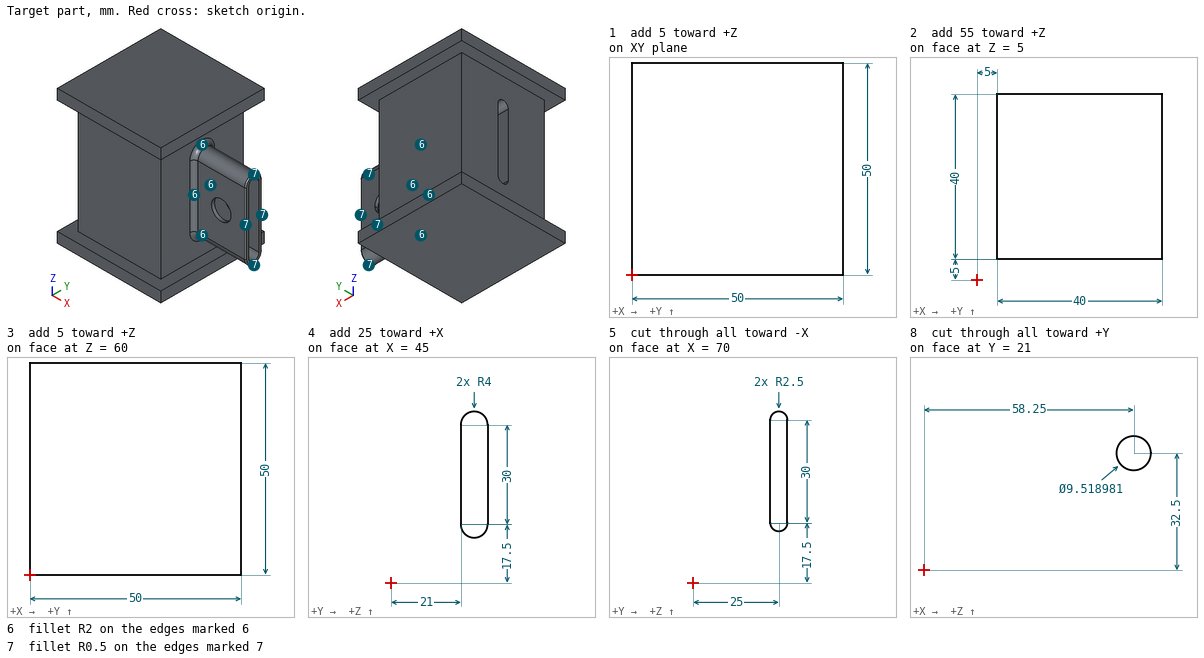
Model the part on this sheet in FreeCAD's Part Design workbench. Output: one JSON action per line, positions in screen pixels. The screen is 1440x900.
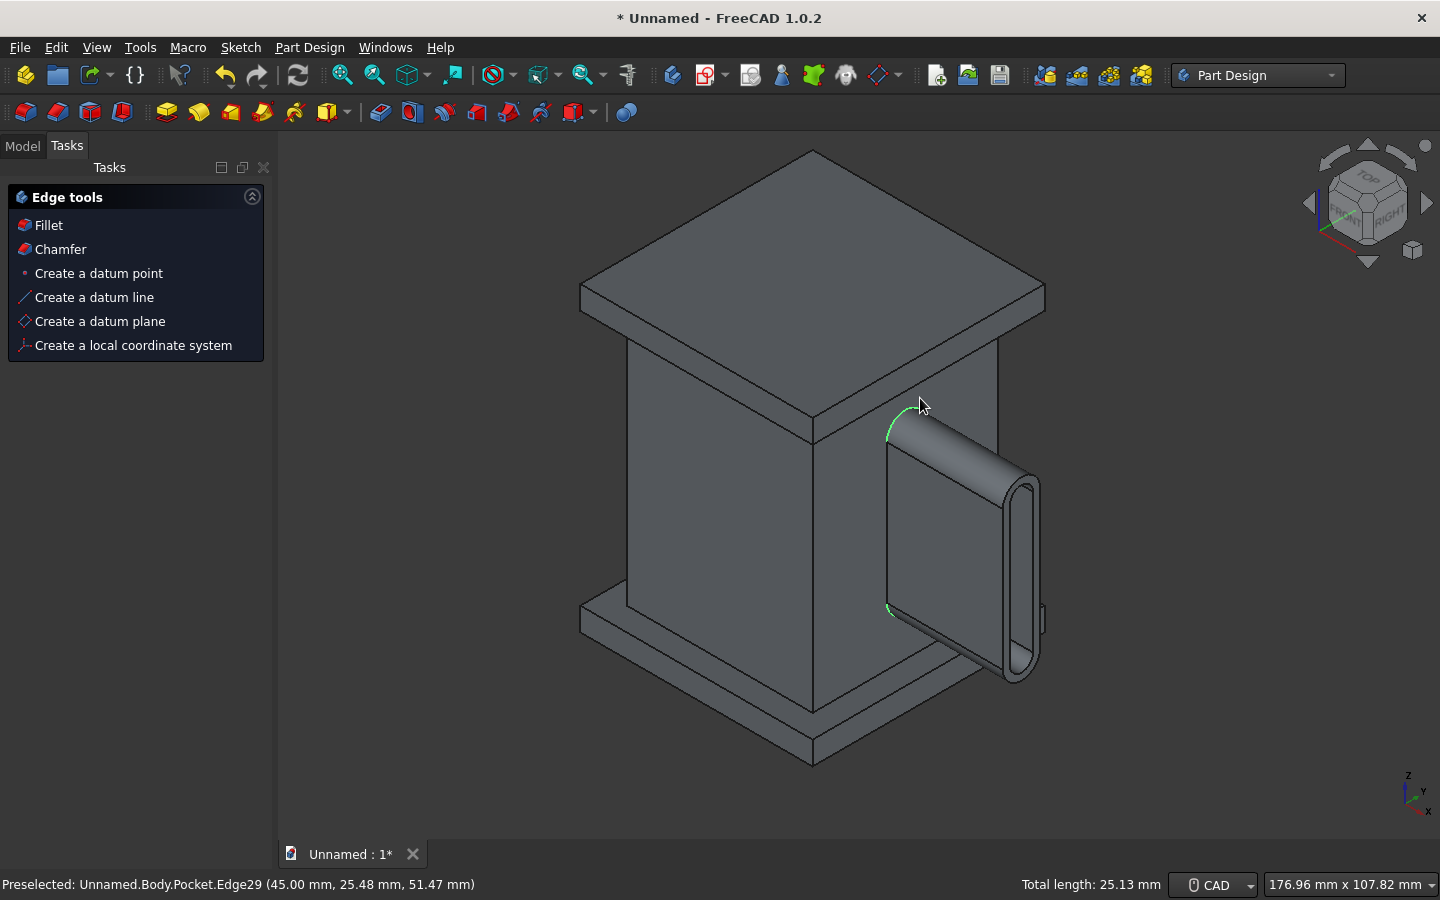
{"action": "key", "text": "2"}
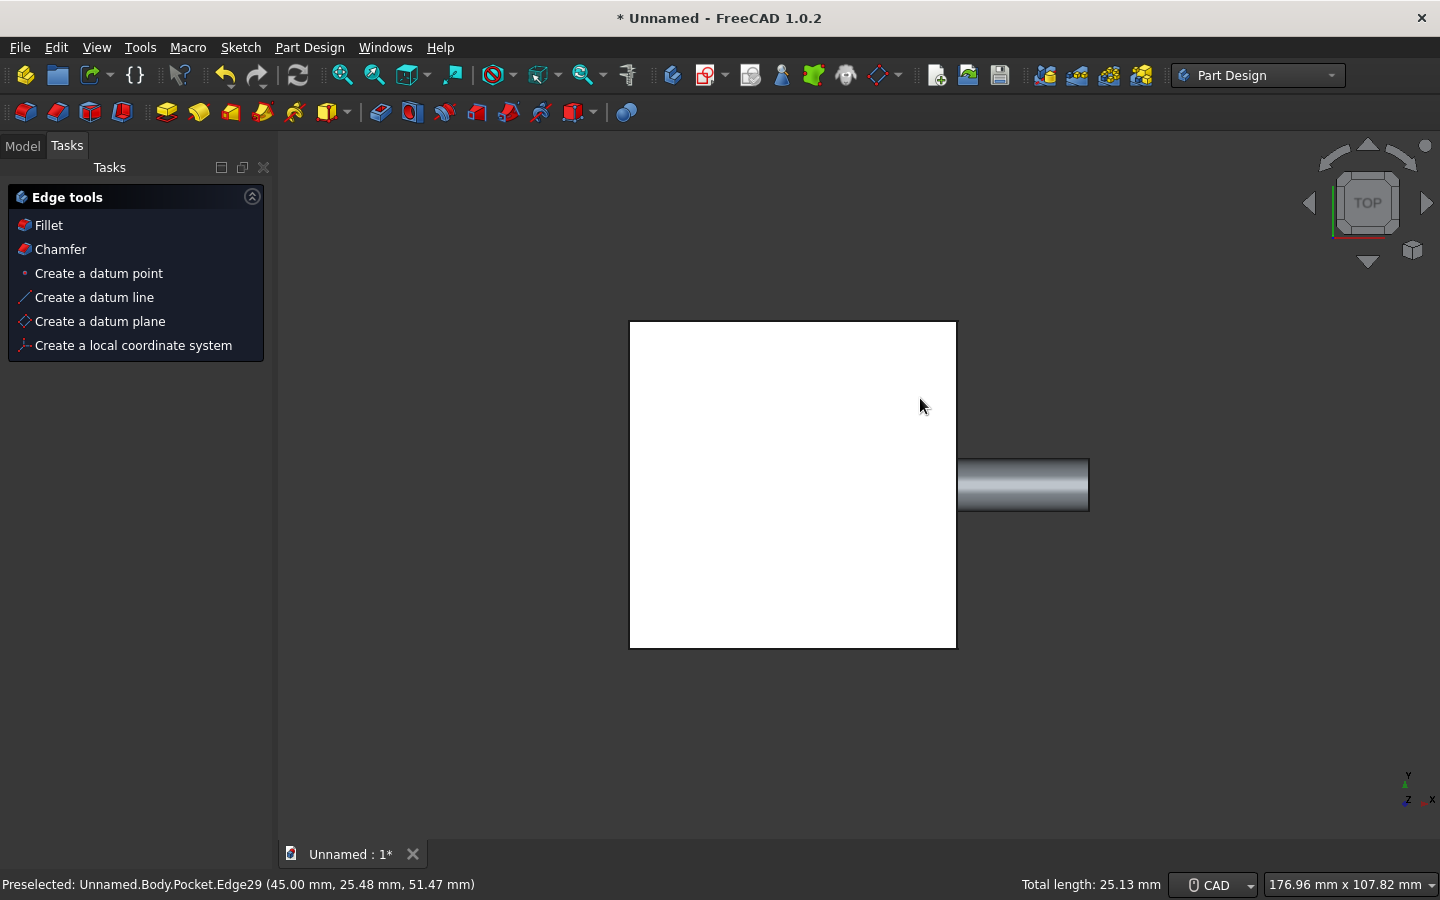
{"action": "key", "text": "1"}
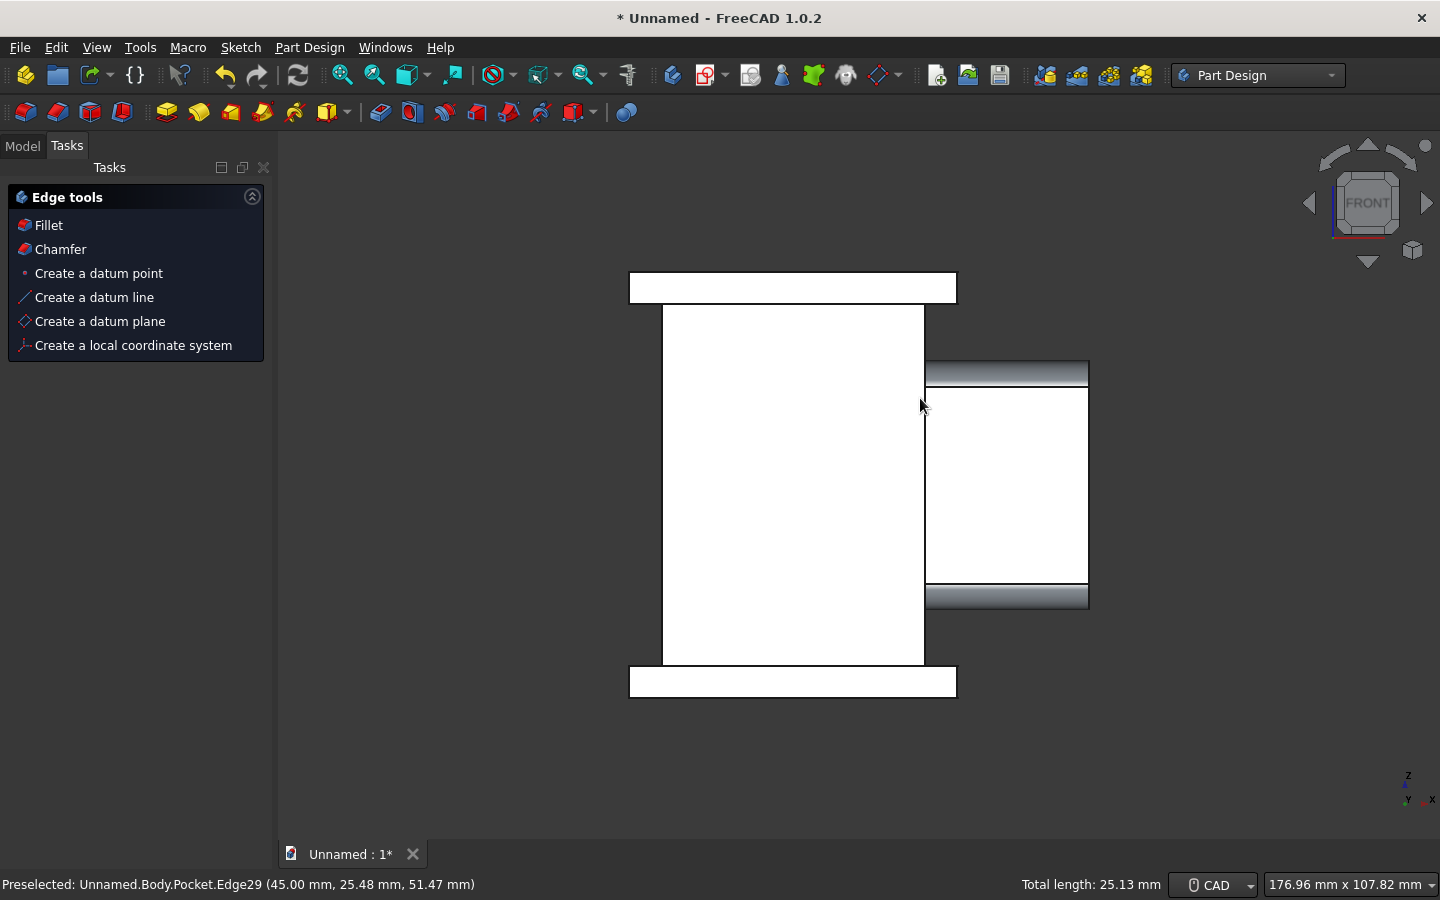
{"action": "key", "text": "3"}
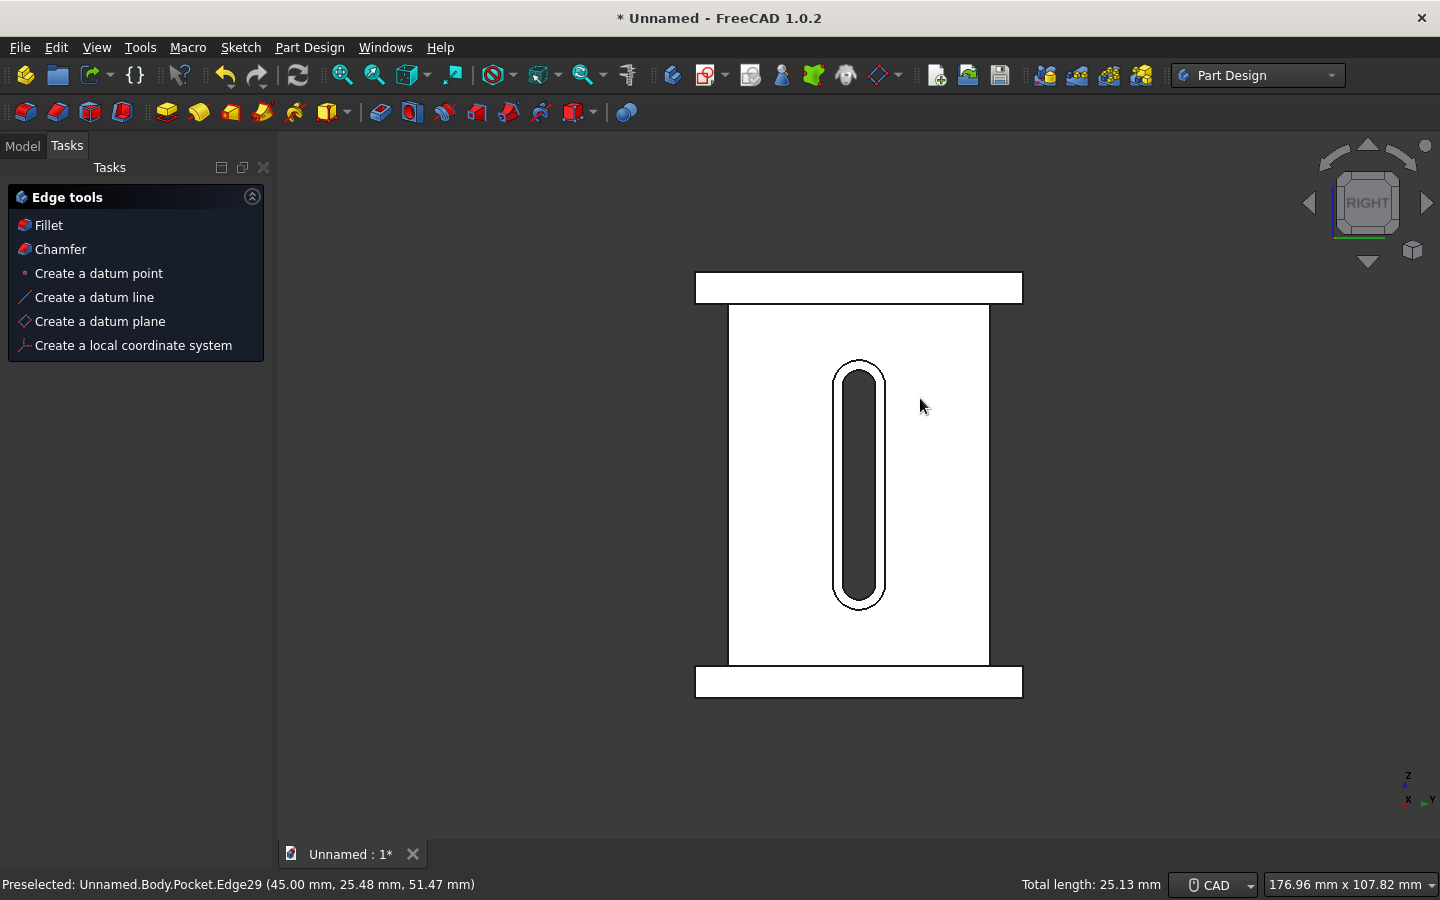
{"action": "key", "text": "5"}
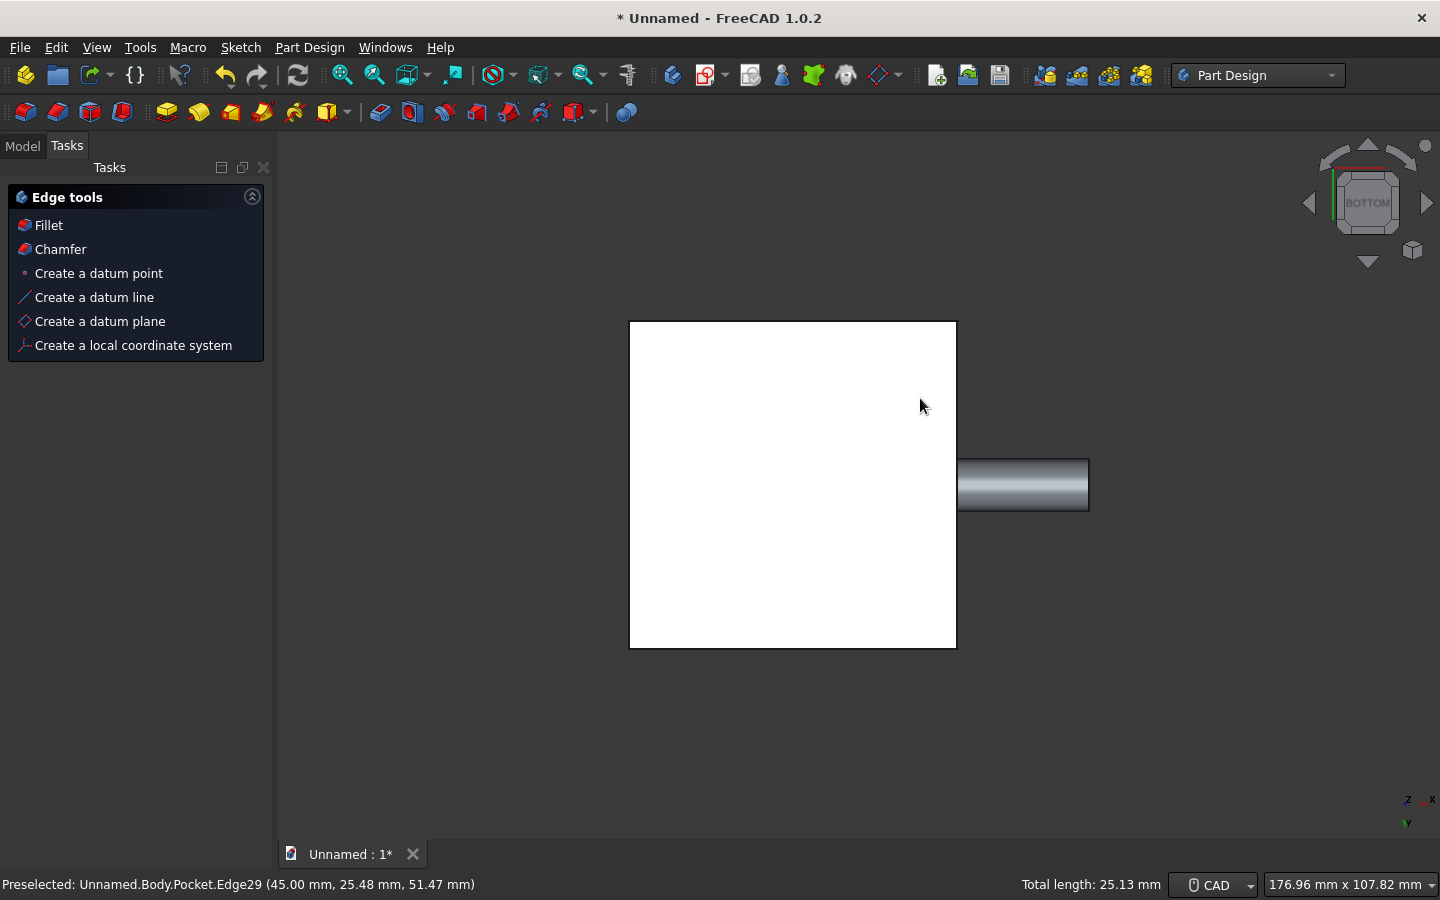
{"action": "key", "text": "4"}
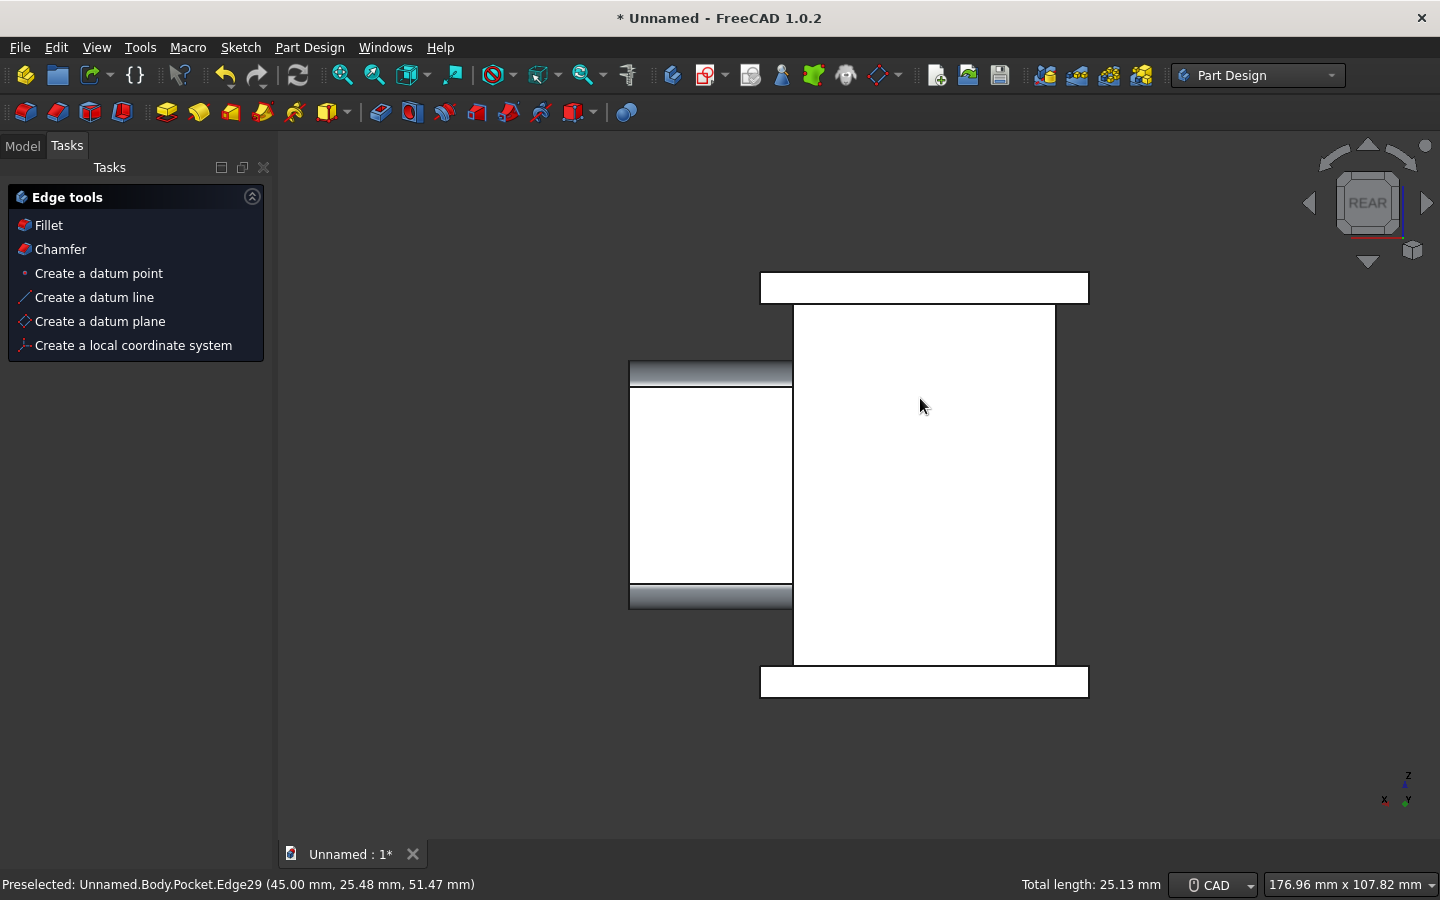
{"action": "key", "text": "6"}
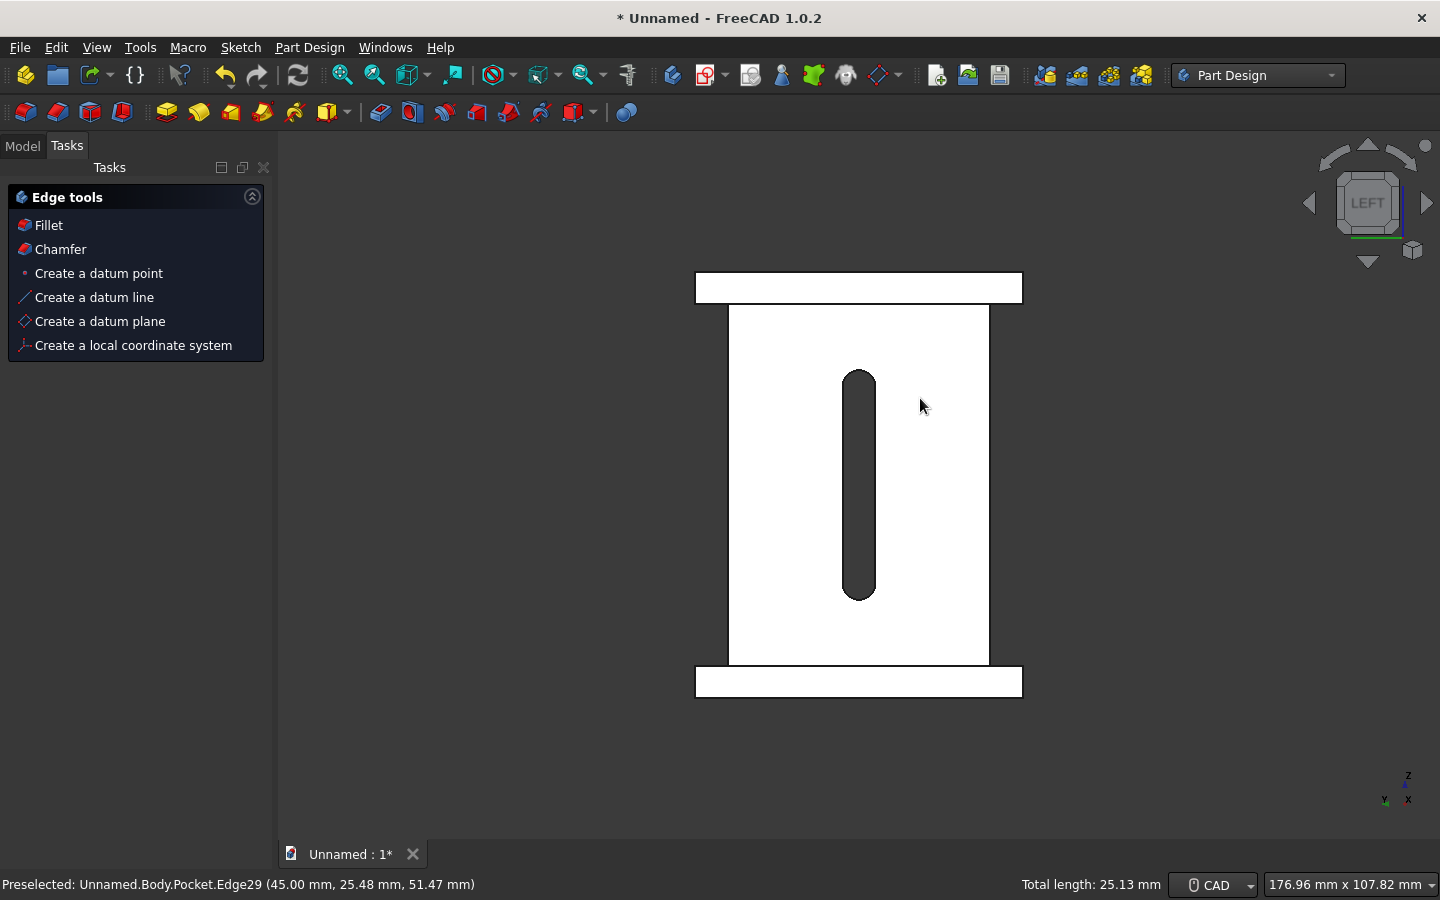
{"action": "key", "text": "v 3"}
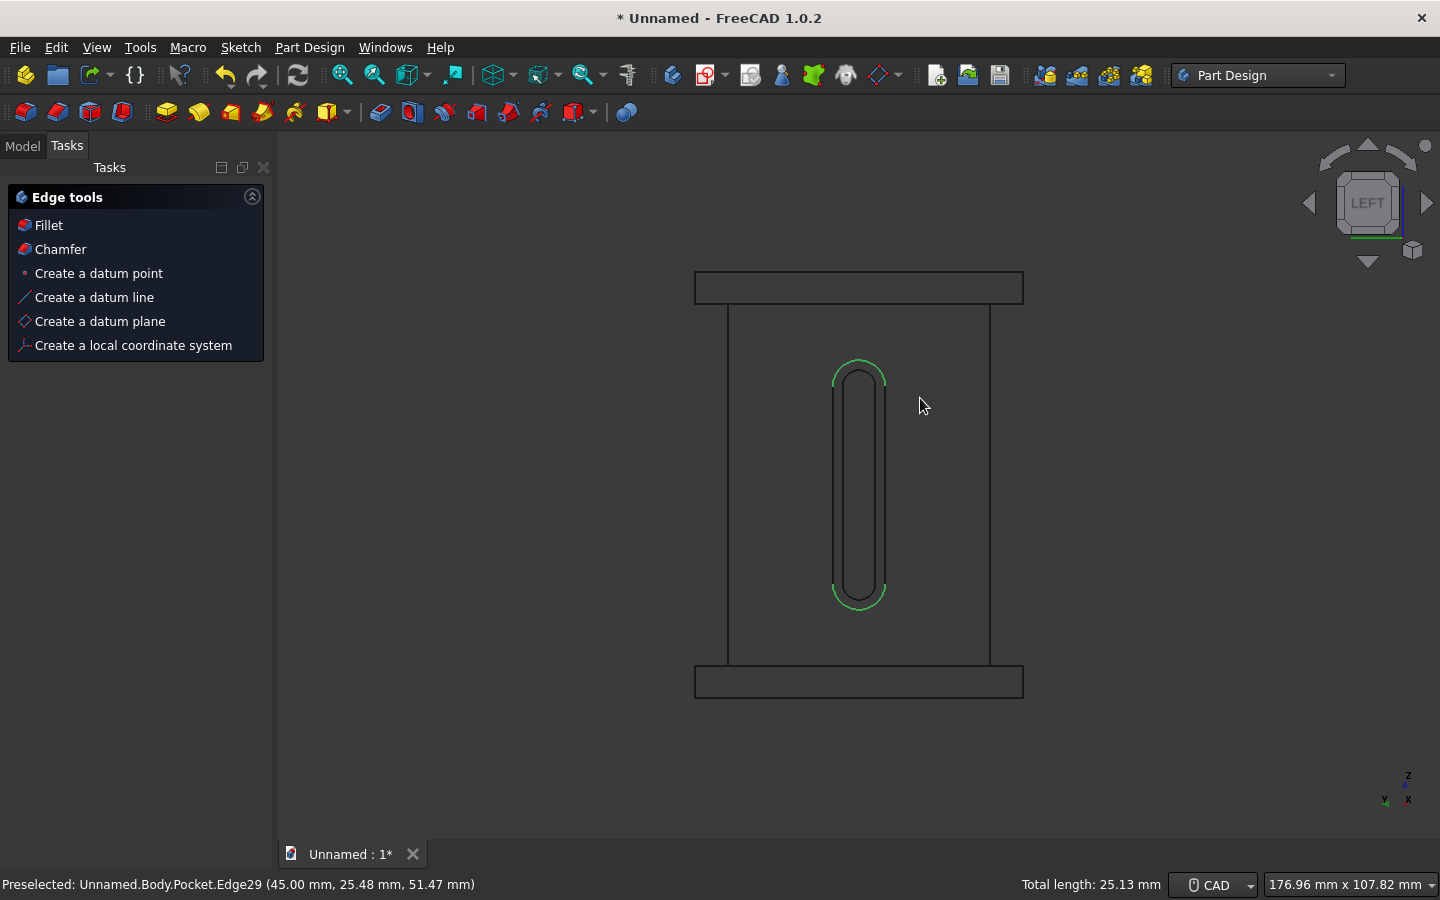
{"action": "key", "text": "0"}